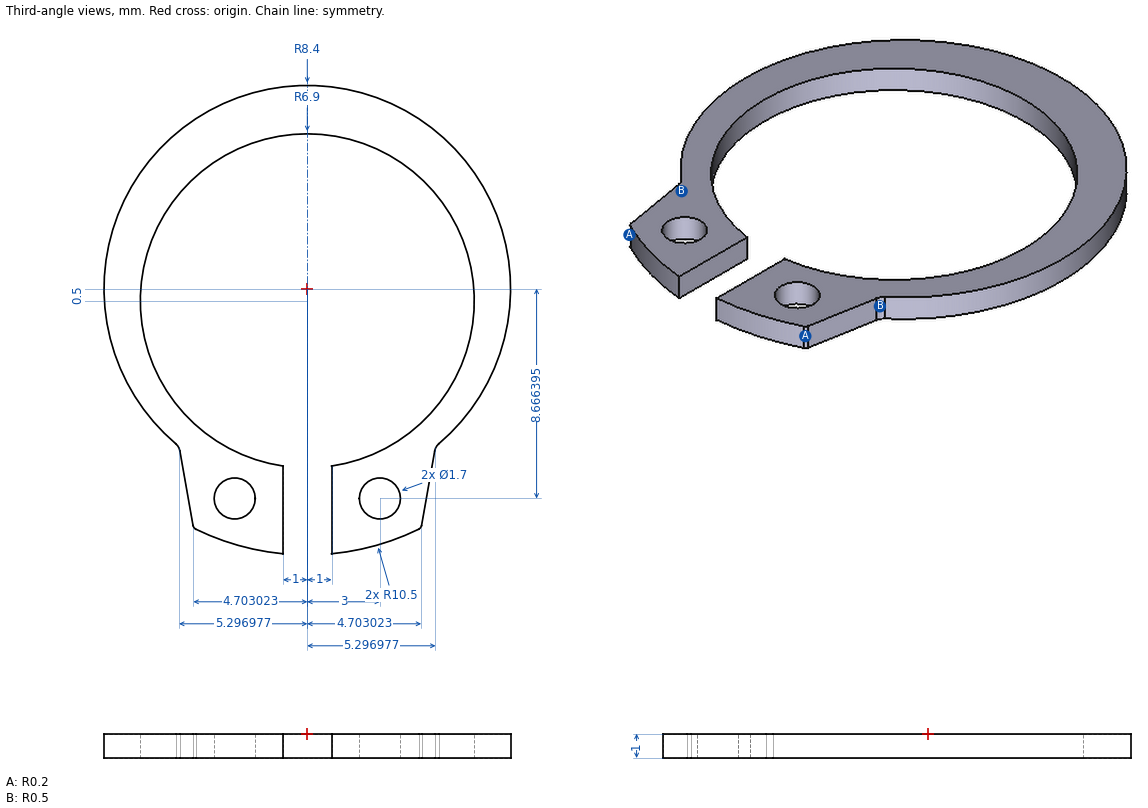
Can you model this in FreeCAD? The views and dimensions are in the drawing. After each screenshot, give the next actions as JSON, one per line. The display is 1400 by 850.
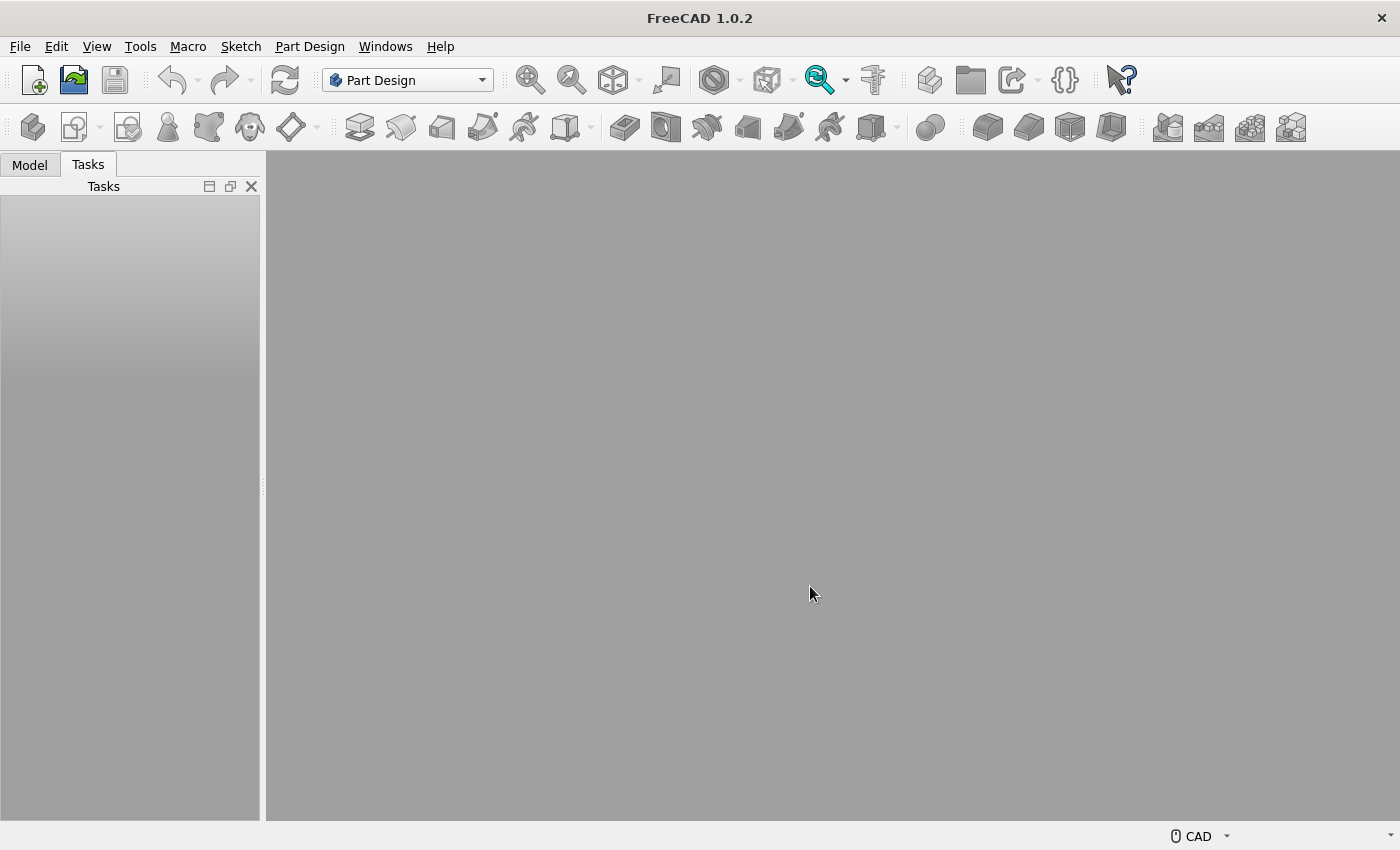
{"action": "left_click", "coordinate": [33, 80]}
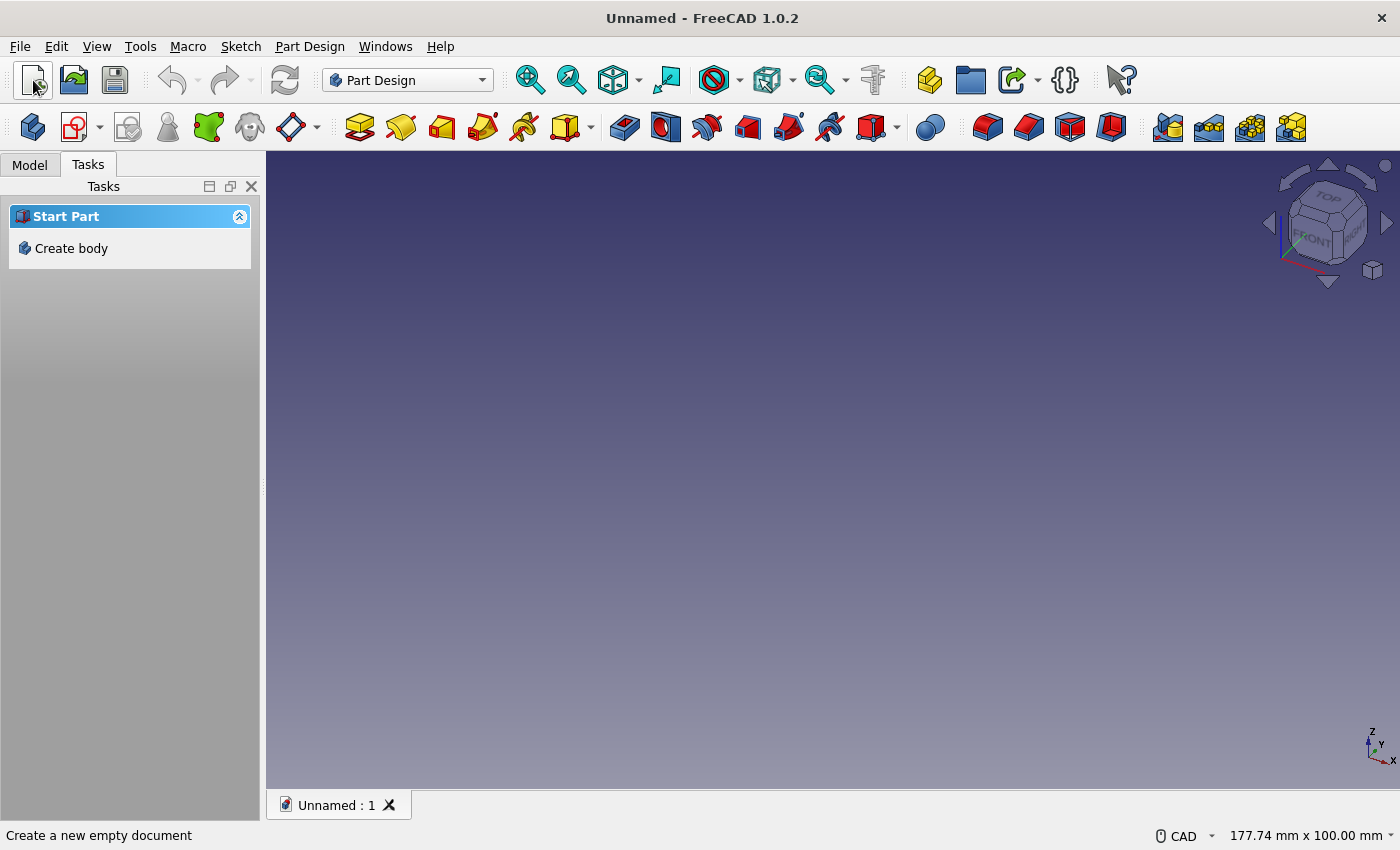
{"action": "left_click", "coordinate": [74, 128]}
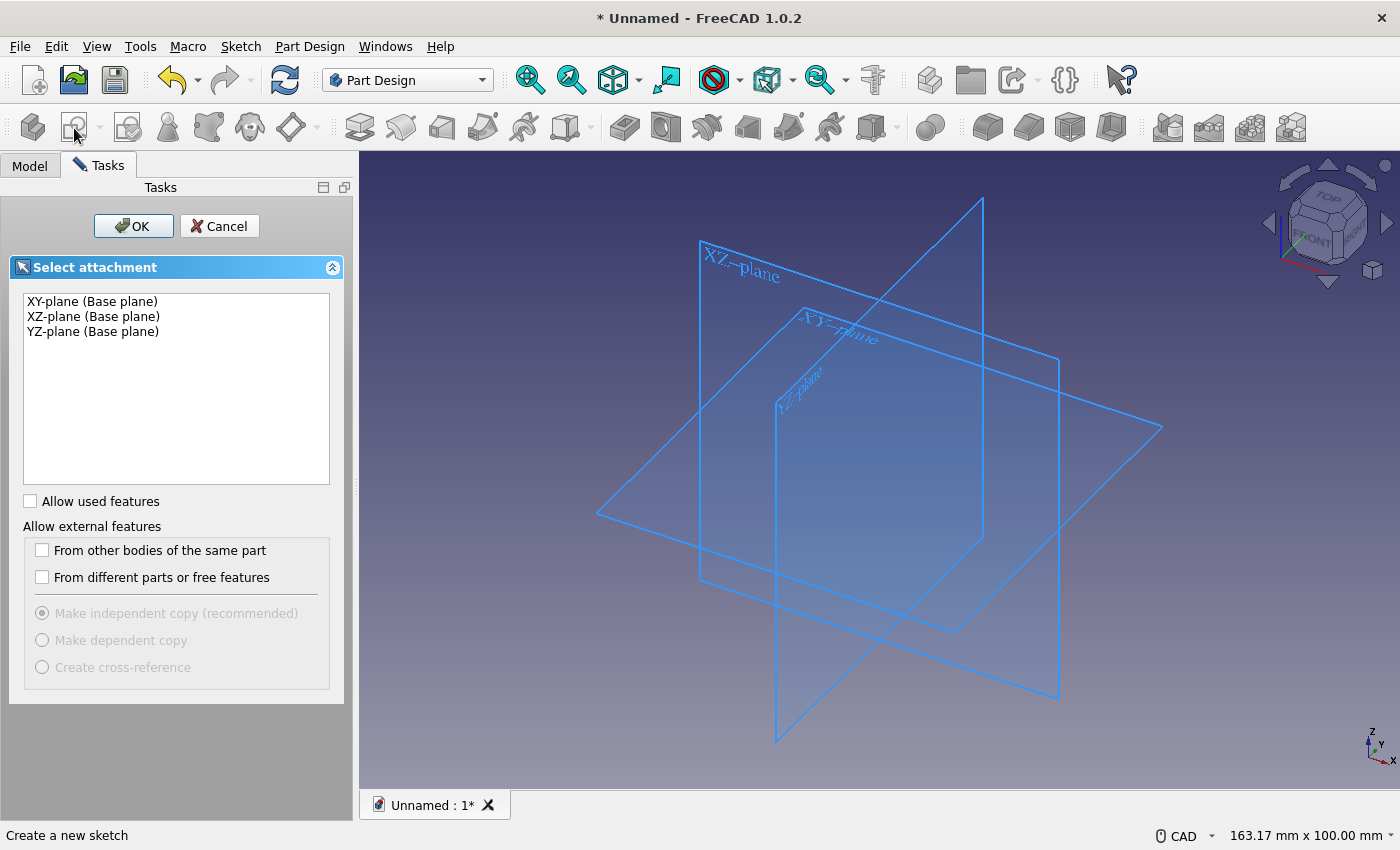
{"action": "left_click", "coordinate": [84, 302]}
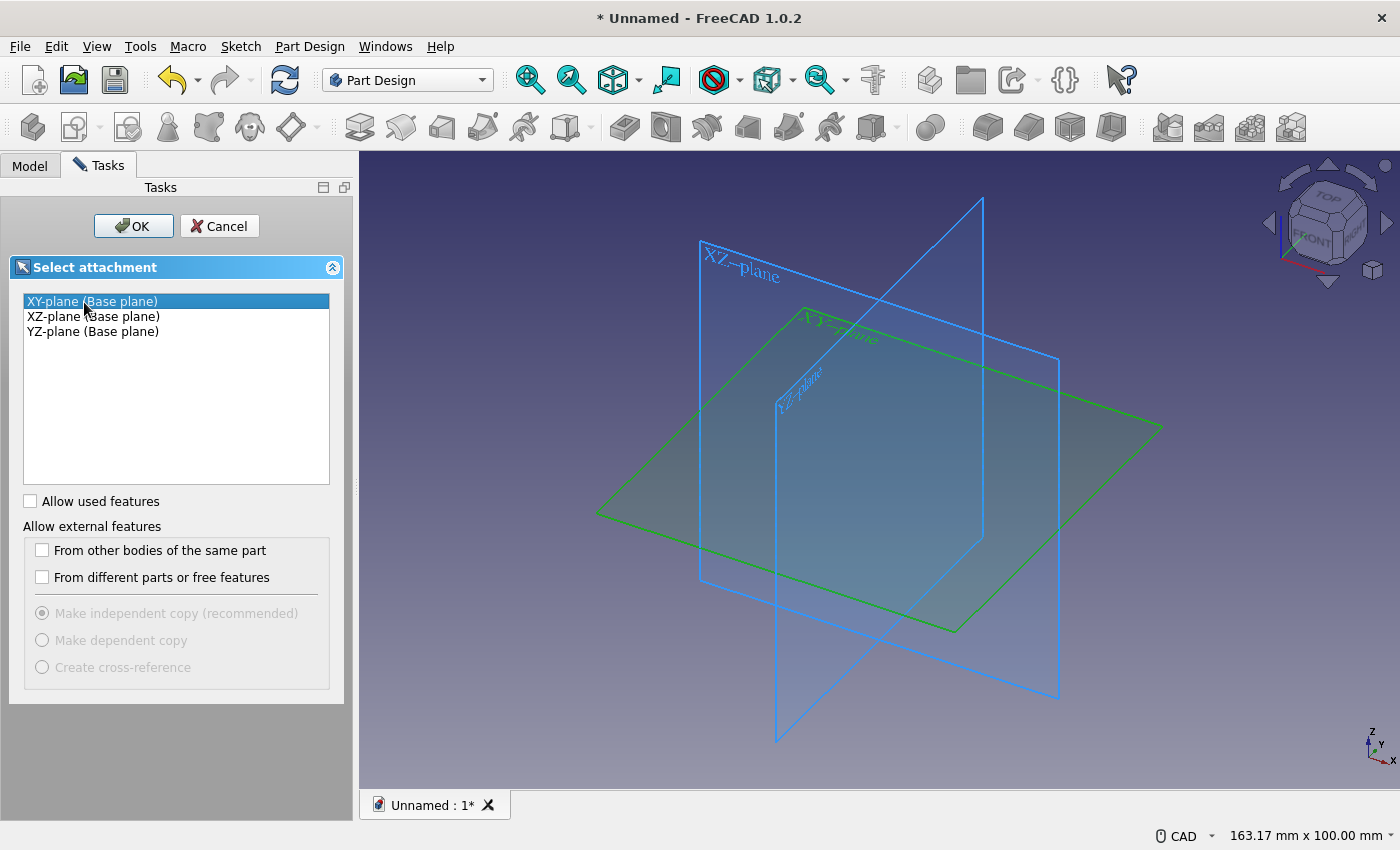
{"action": "left_click", "coordinate": [134, 226]}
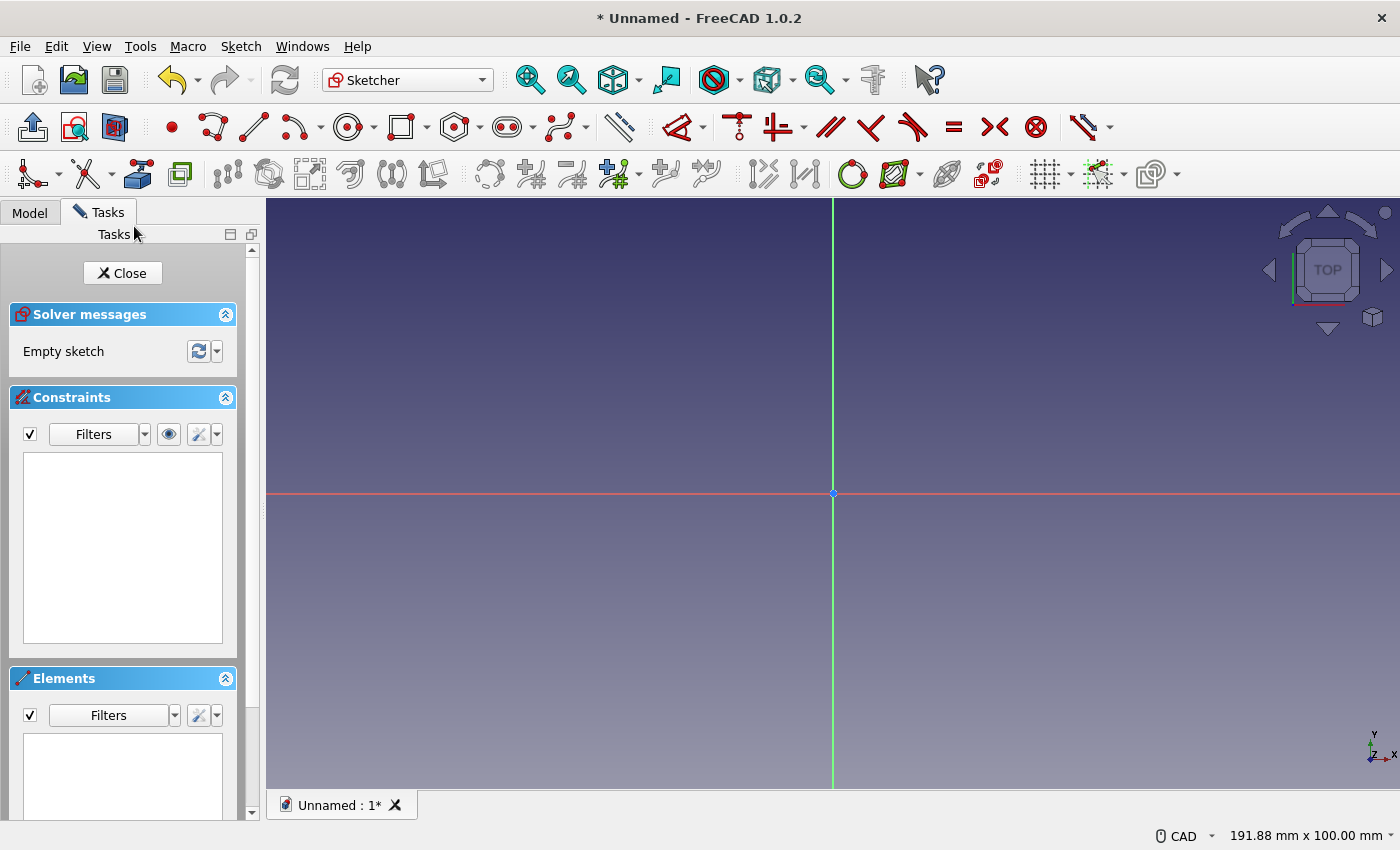
{"action": "scroll", "coordinate": [863, 504], "scroll_direction": "up", "scroll_amount": 6}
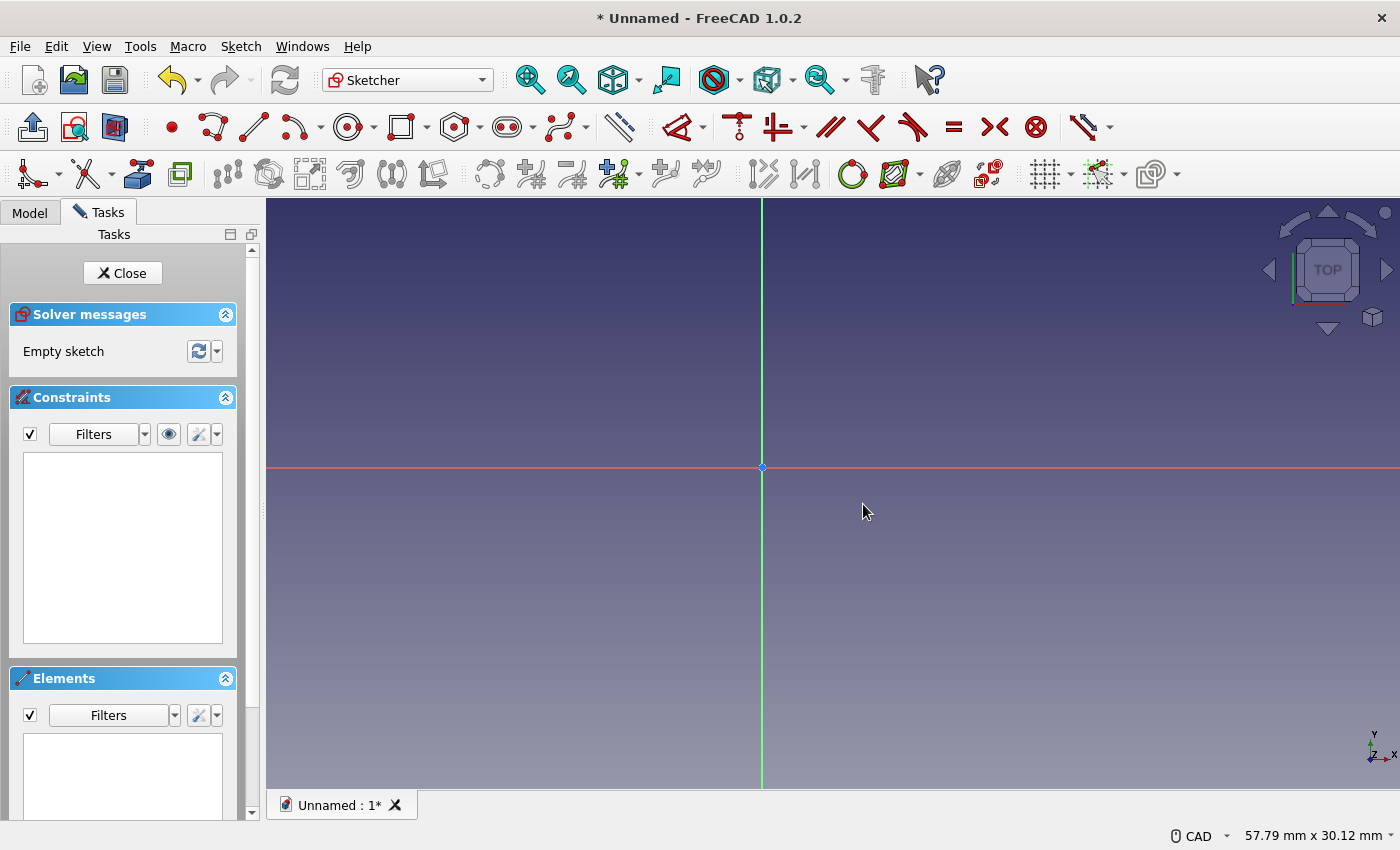
{"action": "left_click", "coordinate": [254, 128]}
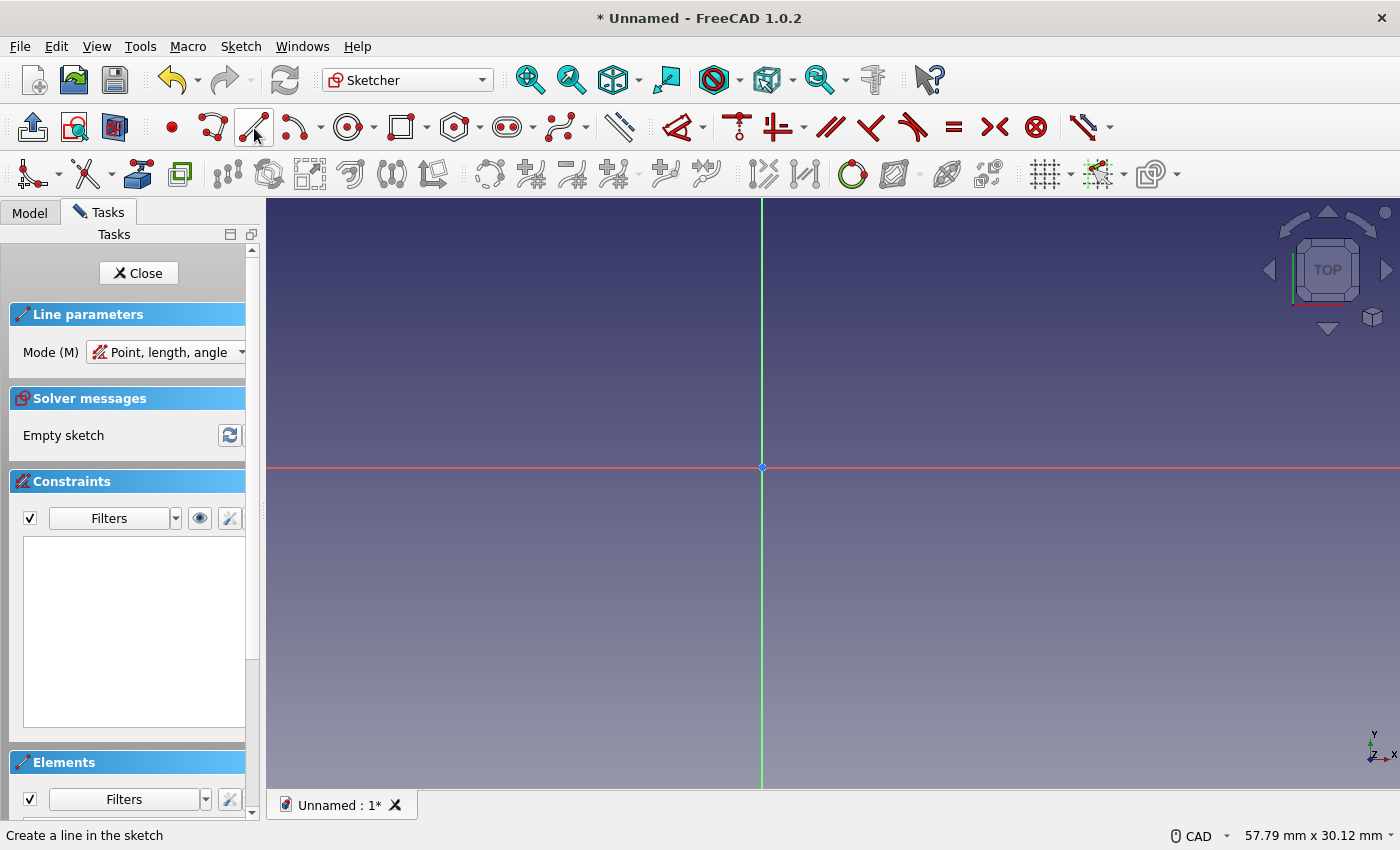
{"action": "left_click", "coordinate": [743, 683]}
{"action": "left_click", "coordinate": [743, 612]}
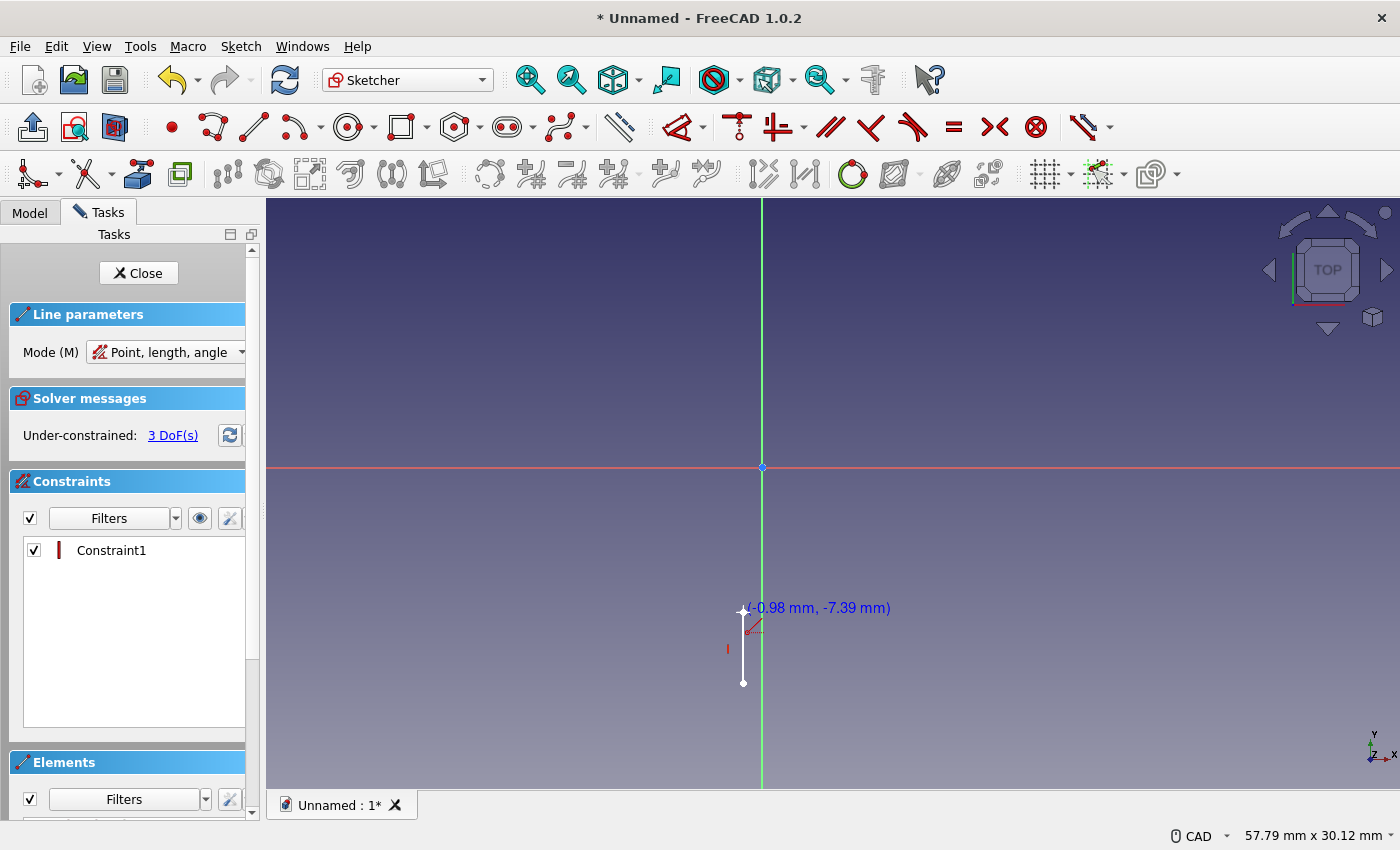
{"action": "left_click", "coordinate": [782, 612]}
{"action": "left_click", "coordinate": [782, 683]}